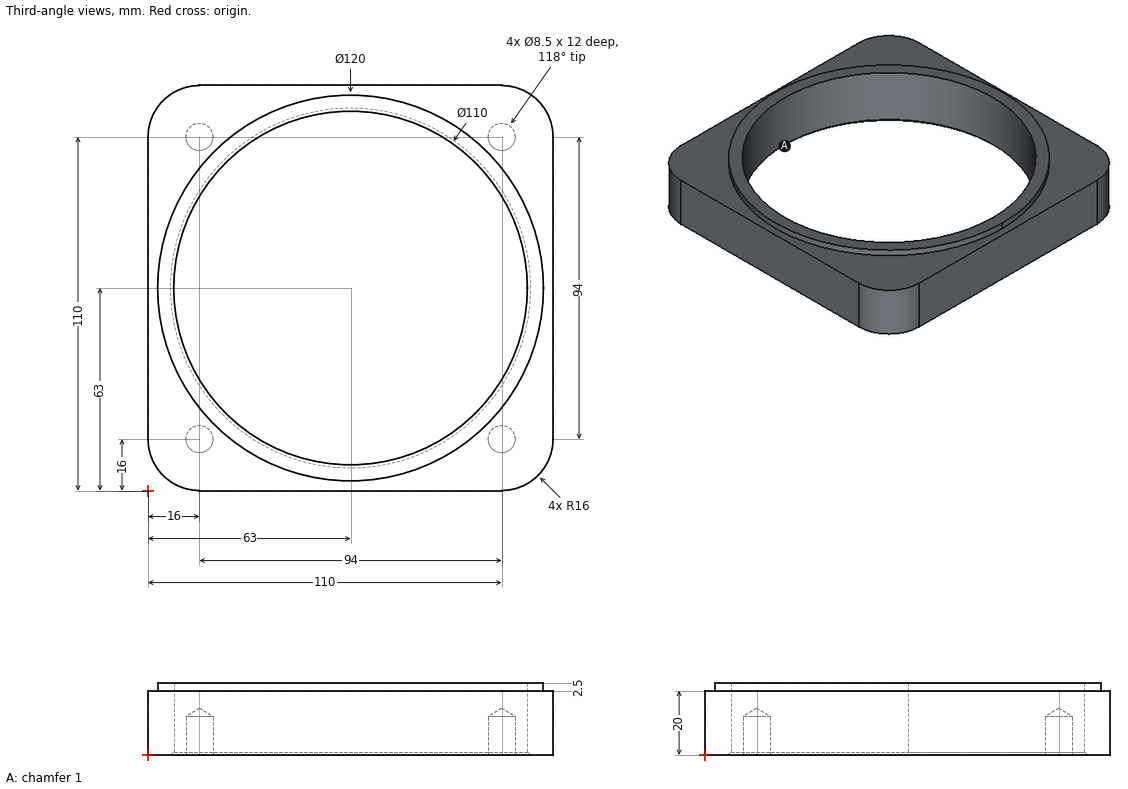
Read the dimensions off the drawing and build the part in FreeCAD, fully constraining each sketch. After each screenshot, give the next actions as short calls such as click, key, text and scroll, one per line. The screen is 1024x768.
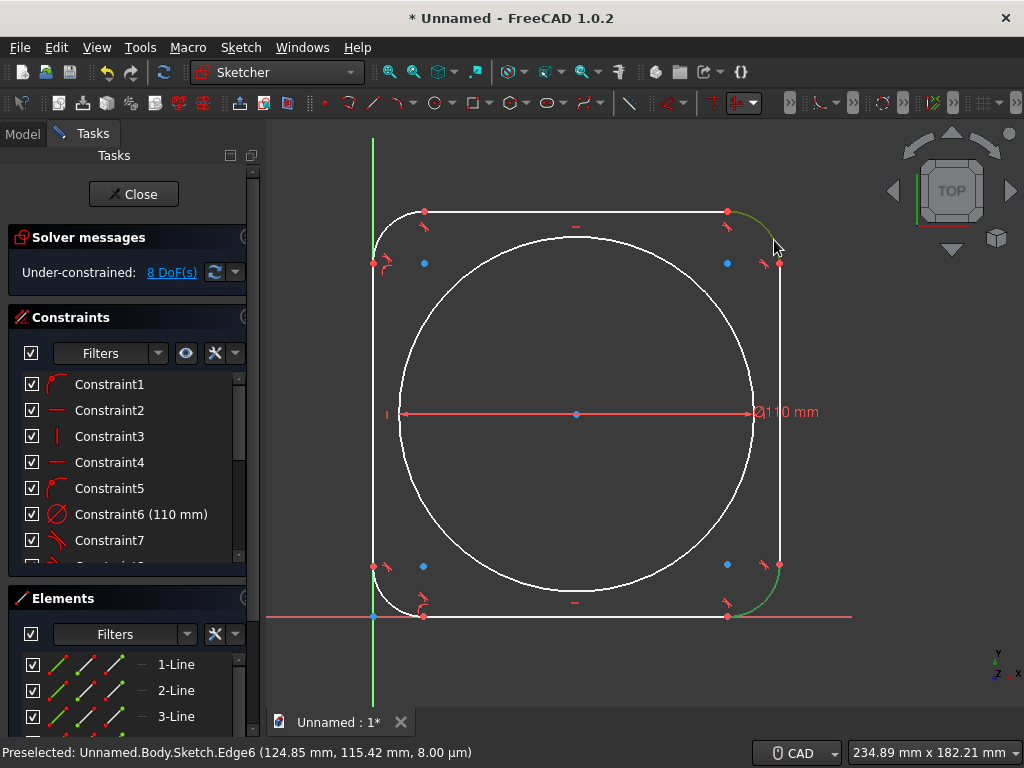
click(401, 217)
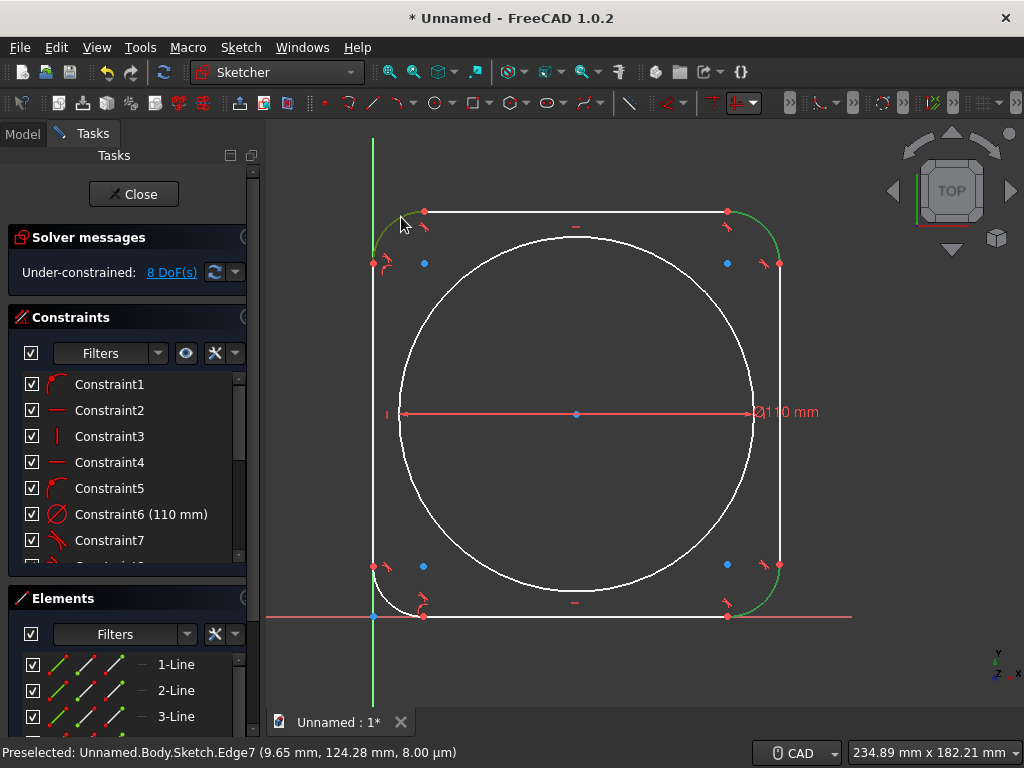
click(388, 602)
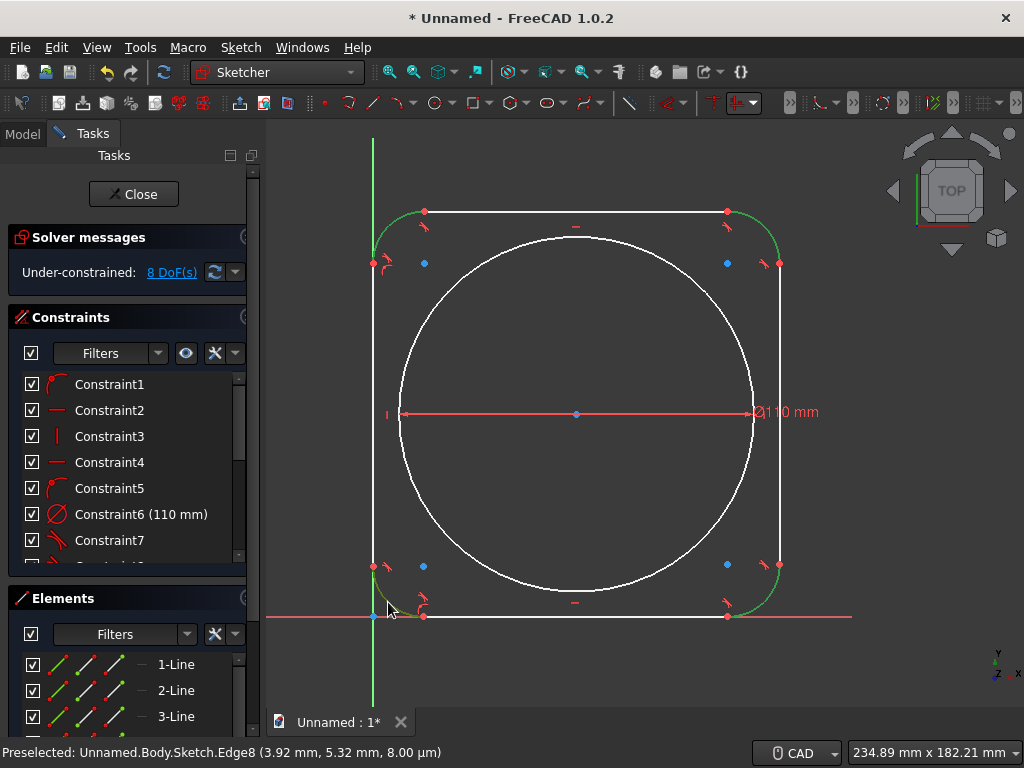
key(e)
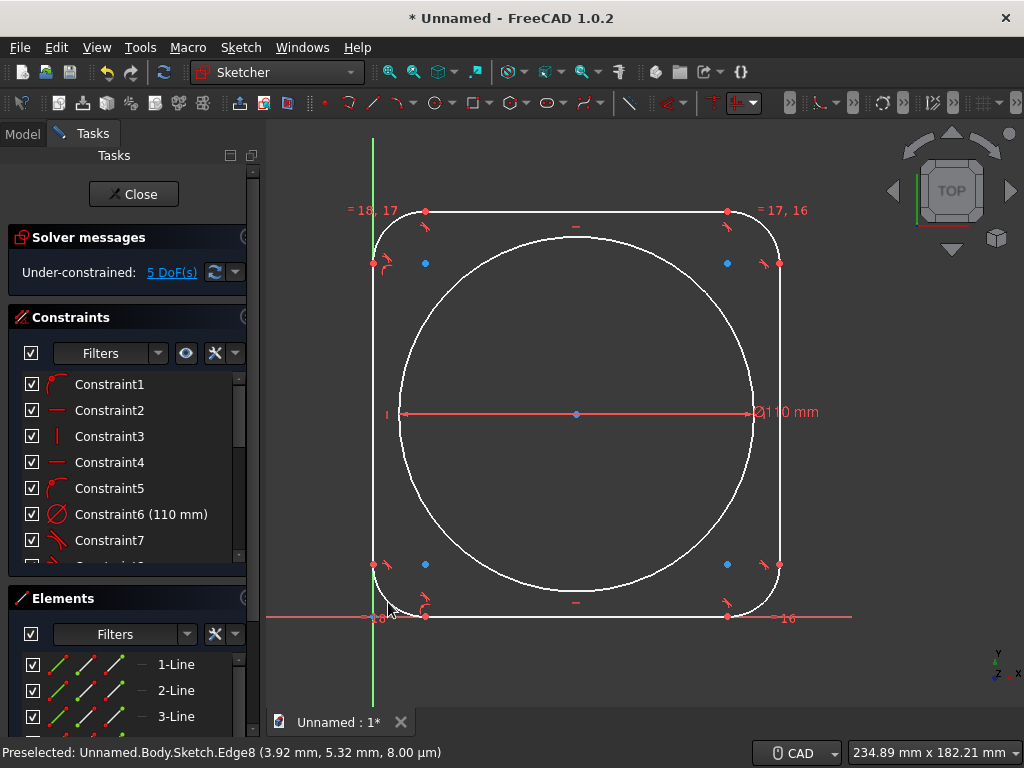
click(774, 589)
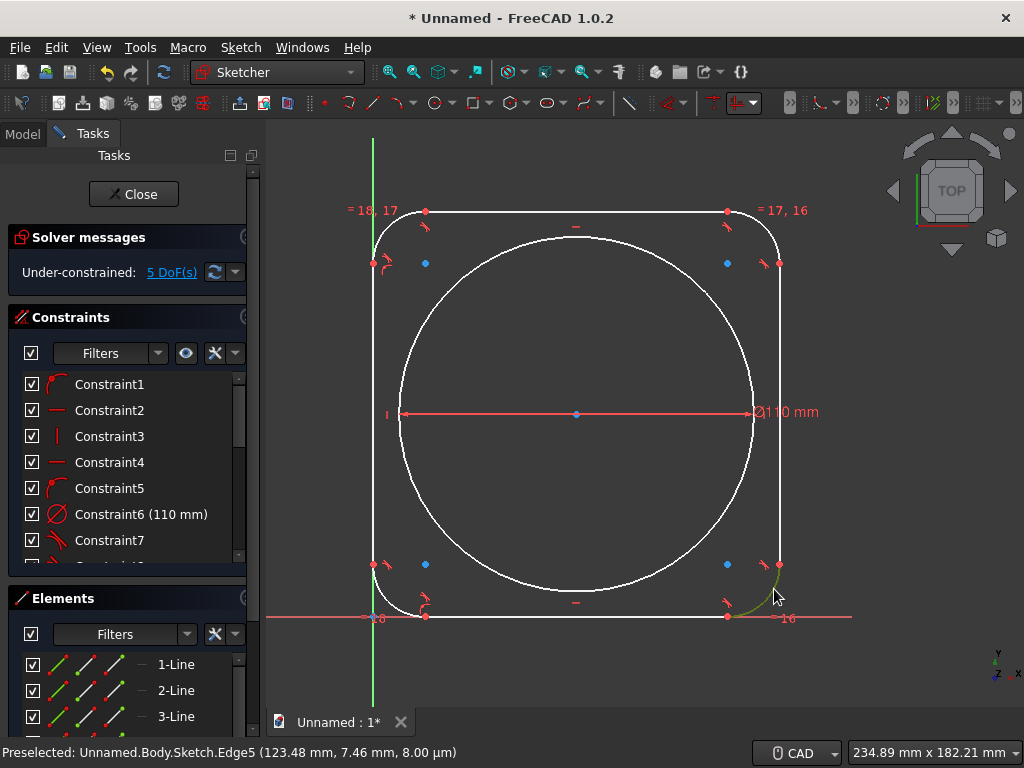
click(686, 104)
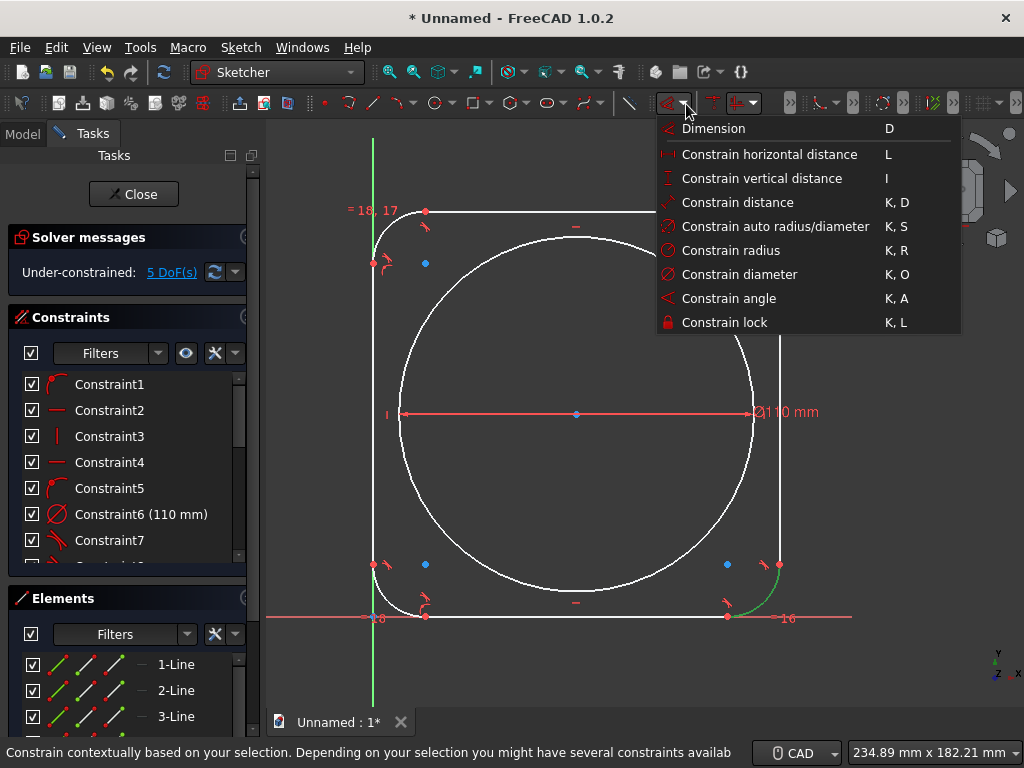
click(809, 250)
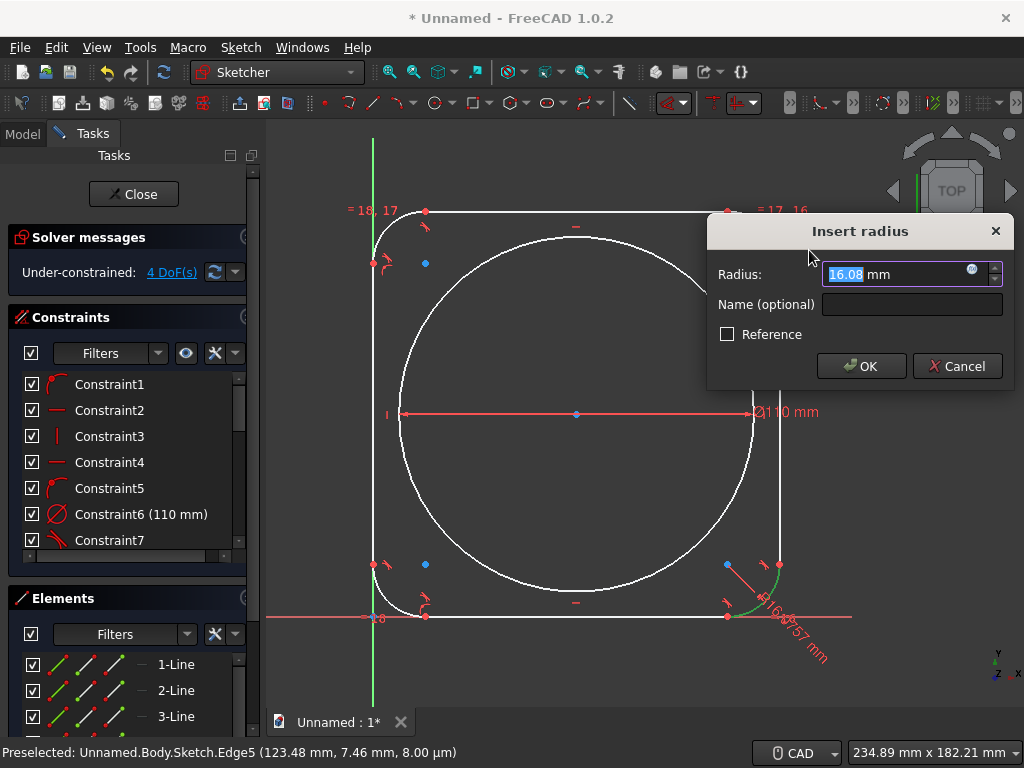
text(16)
key(Return)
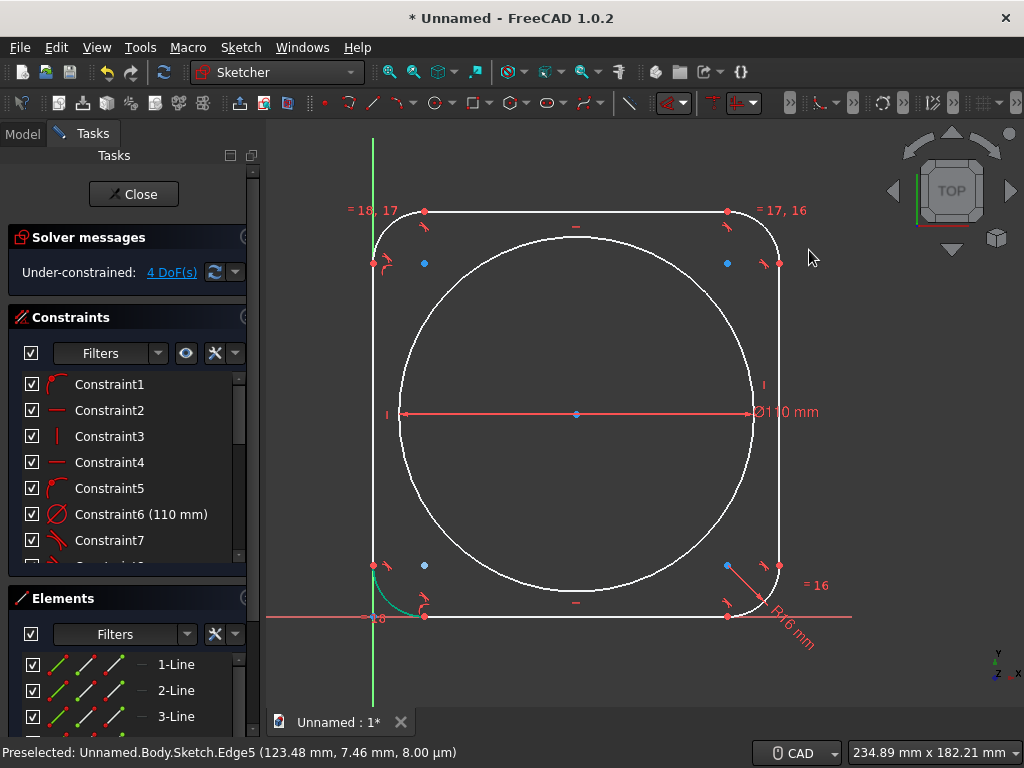
click(516, 617)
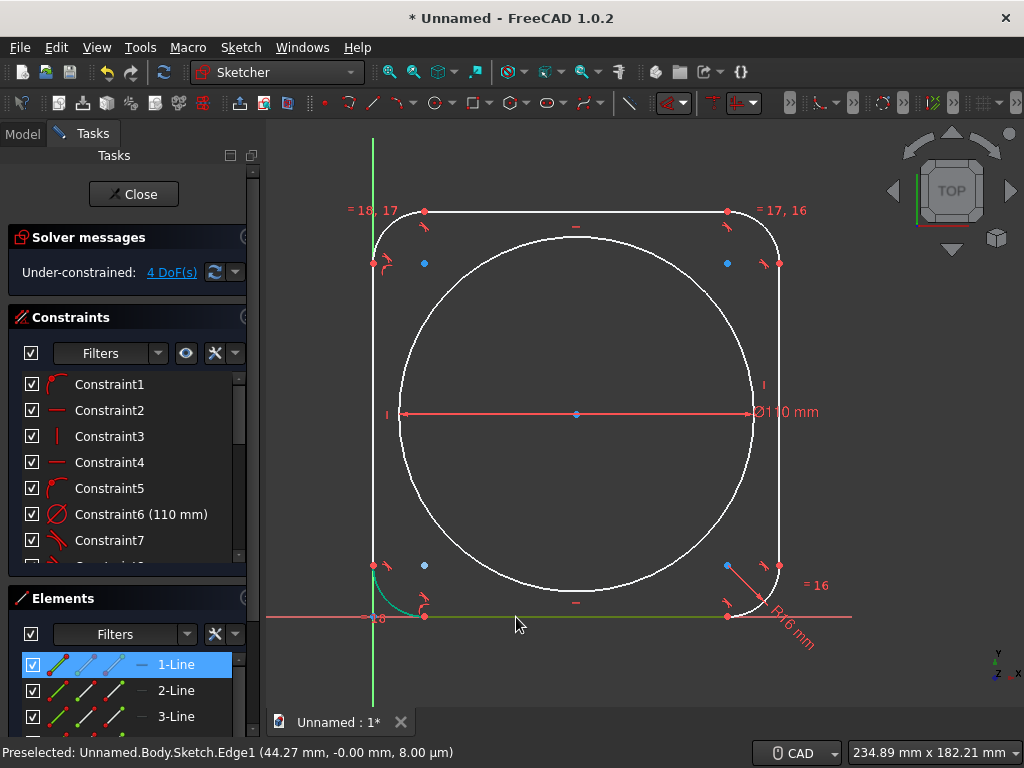
click(686, 104)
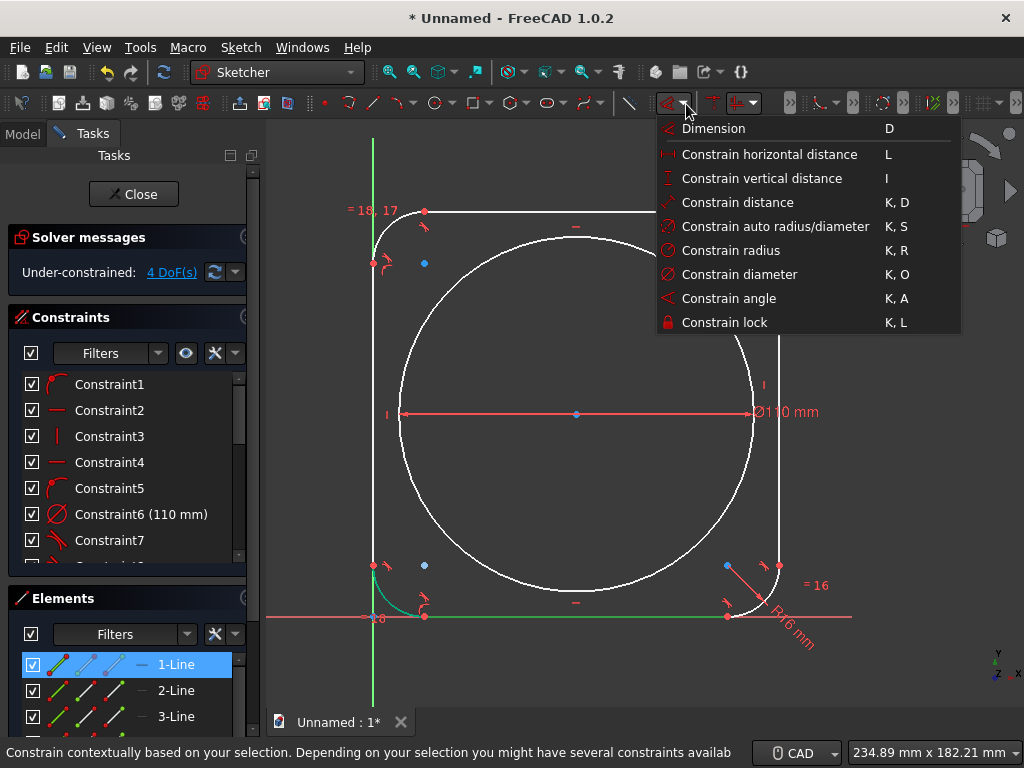
click(809, 154)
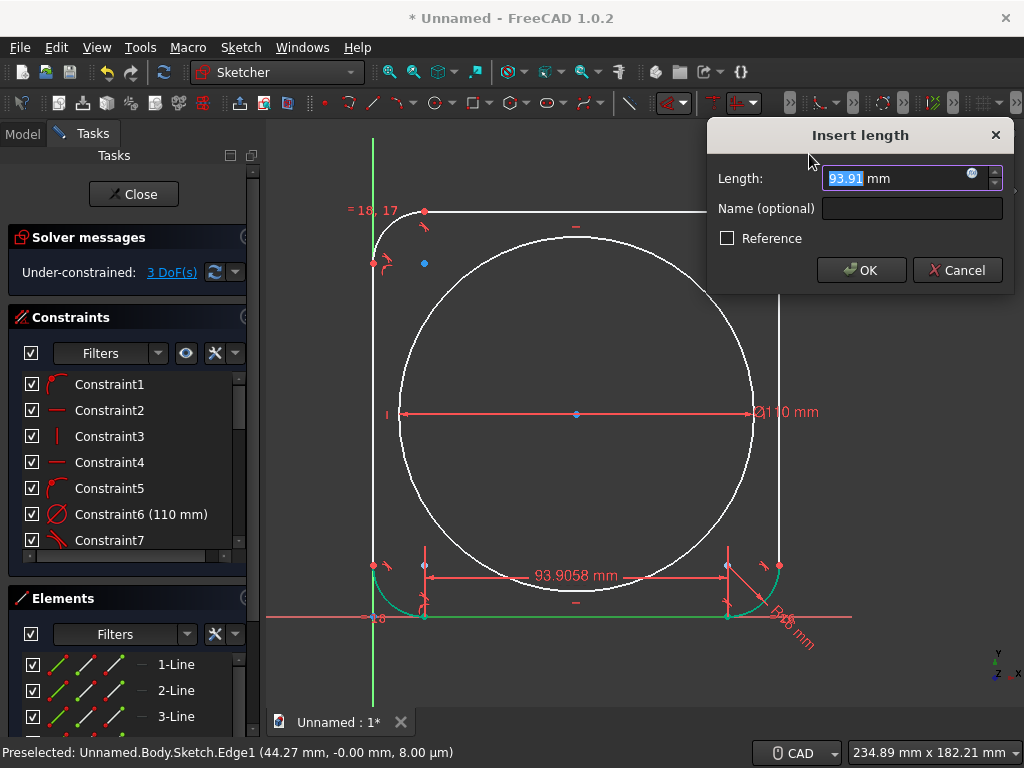
text(94)
key(Return)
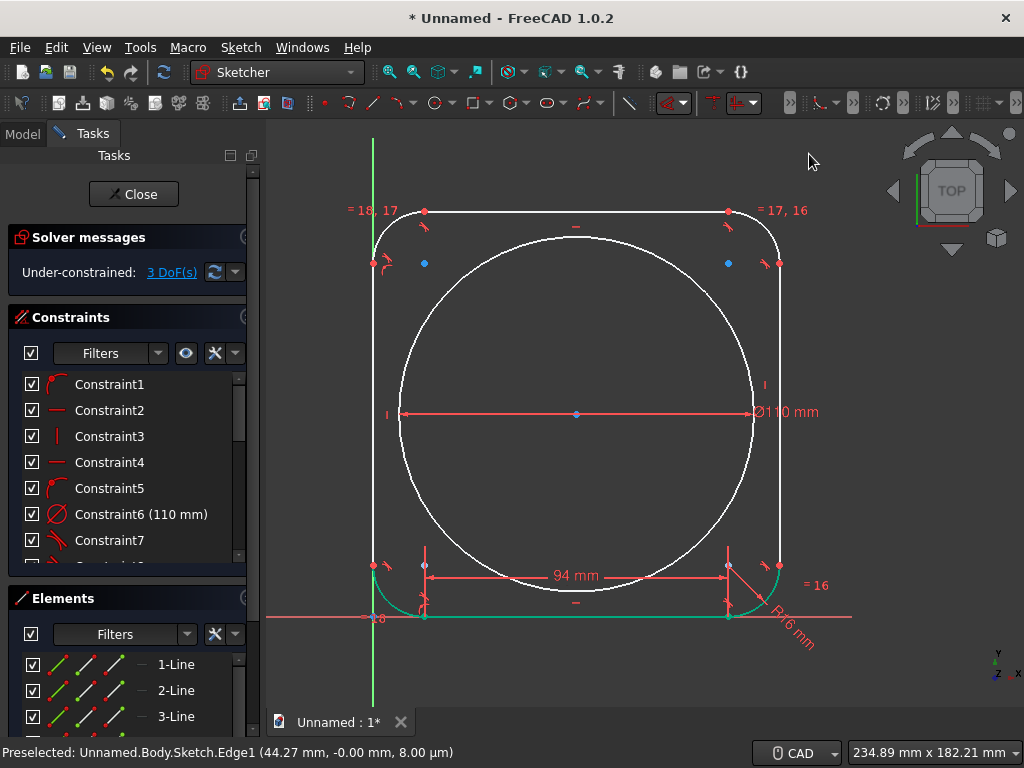
click(780, 475)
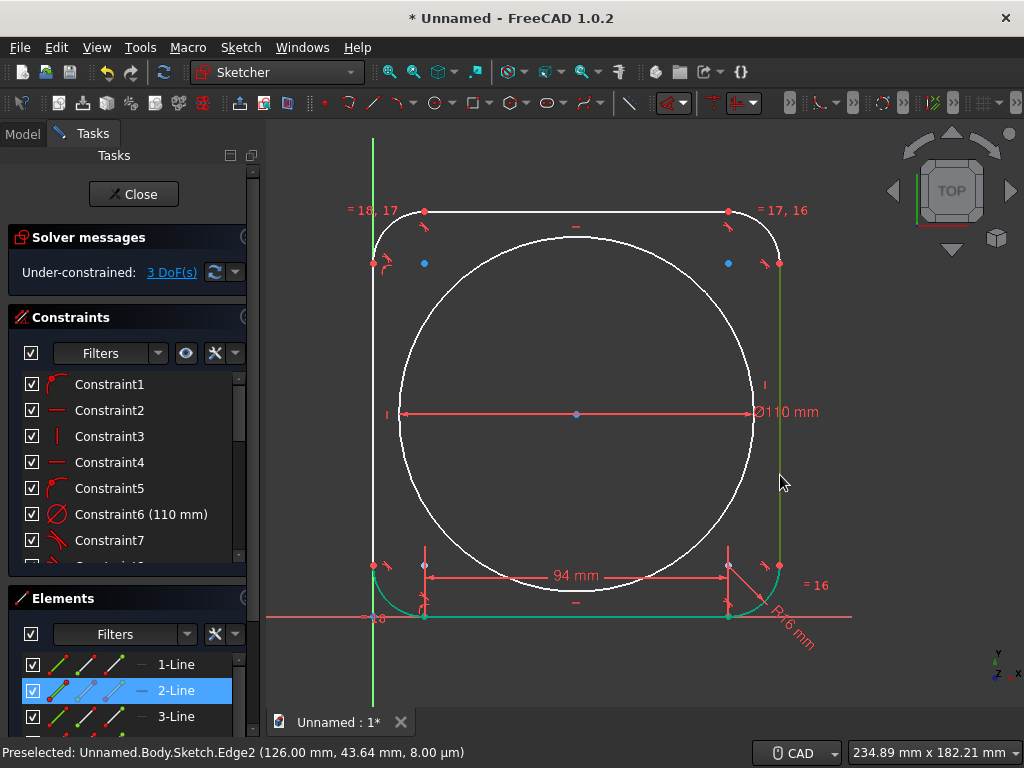
click(686, 104)